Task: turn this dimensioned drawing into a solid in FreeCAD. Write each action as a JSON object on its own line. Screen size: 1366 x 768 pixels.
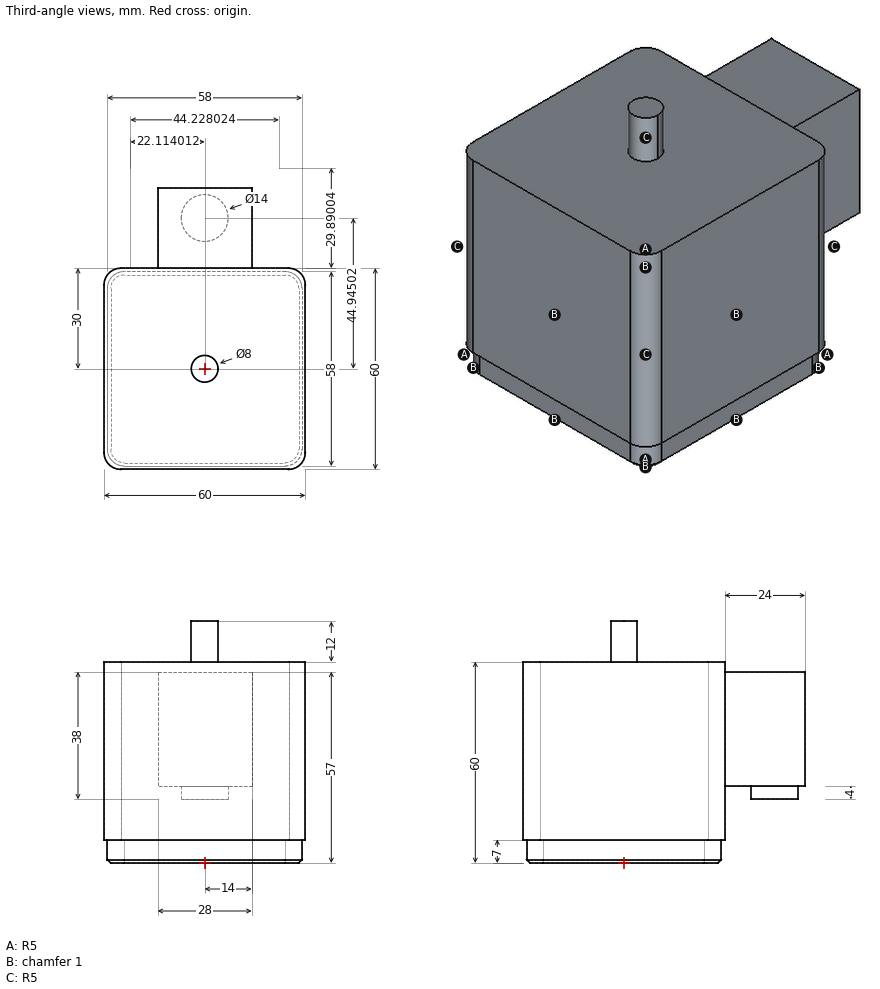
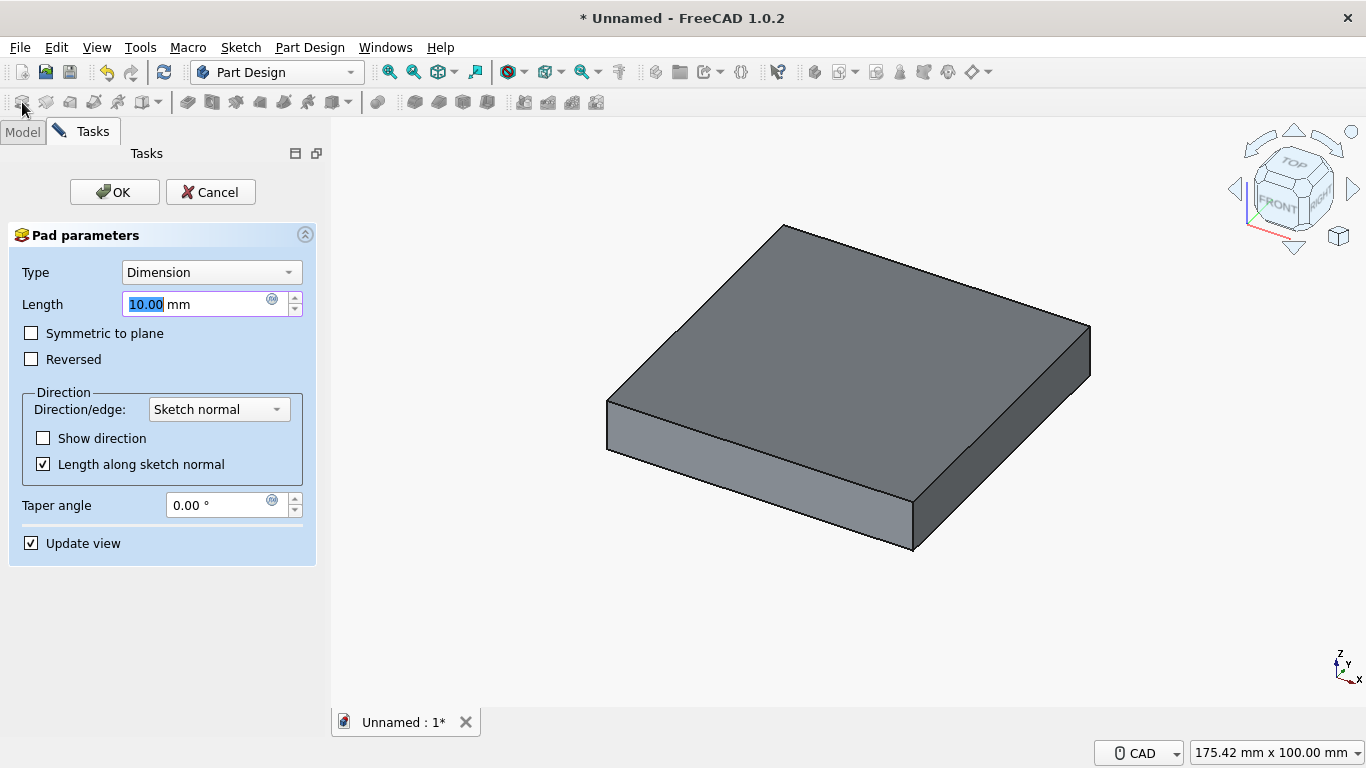
{"action": "type", "text": "60"}
{"action": "key", "text": "Tab"}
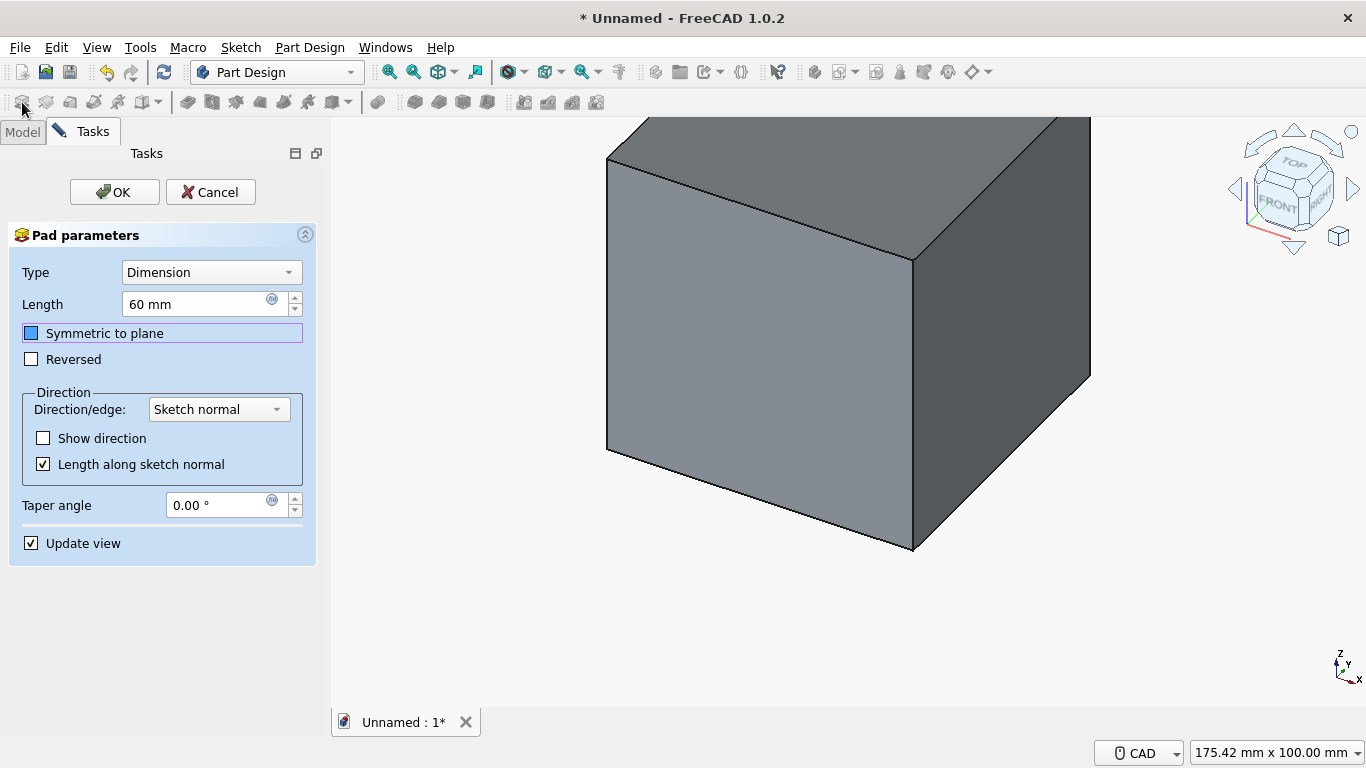
{"action": "left_click", "coordinate": [115, 192]}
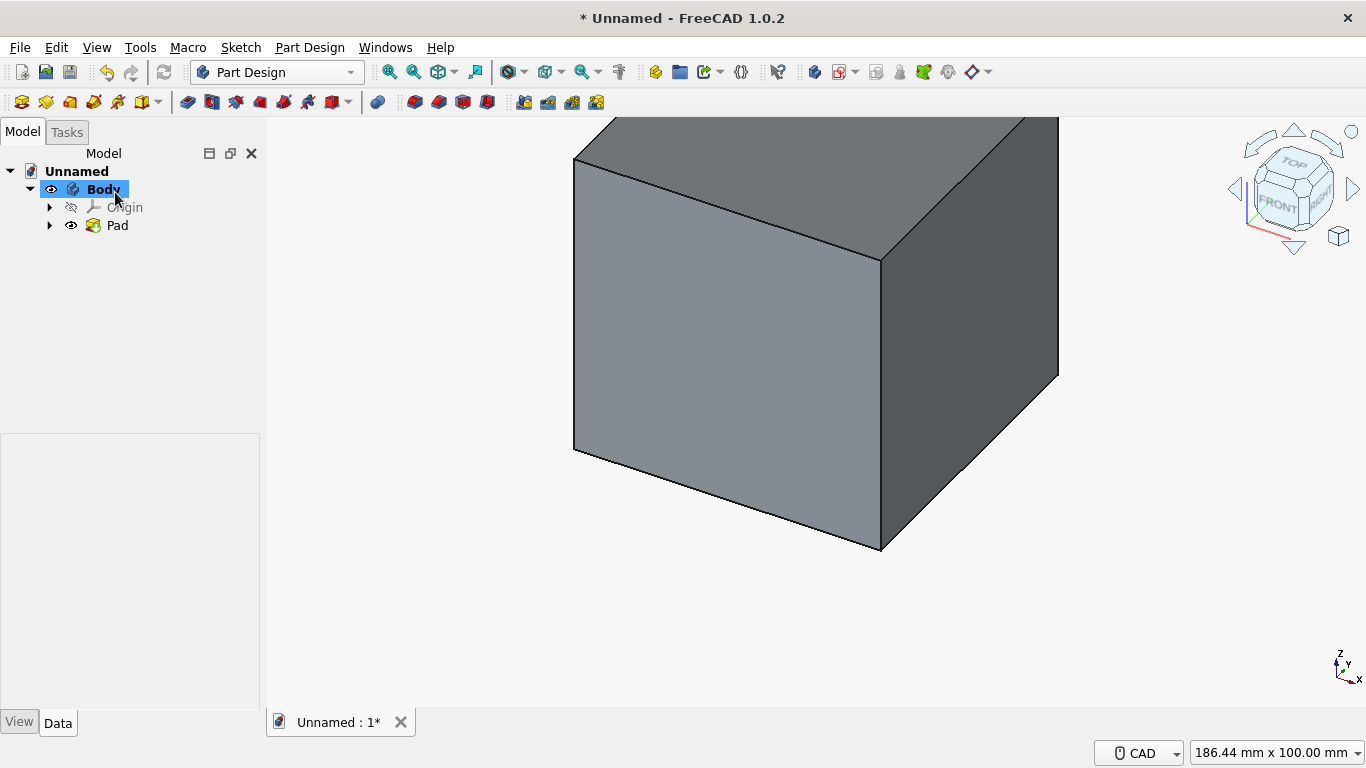
{"action": "key", "text": "v f"}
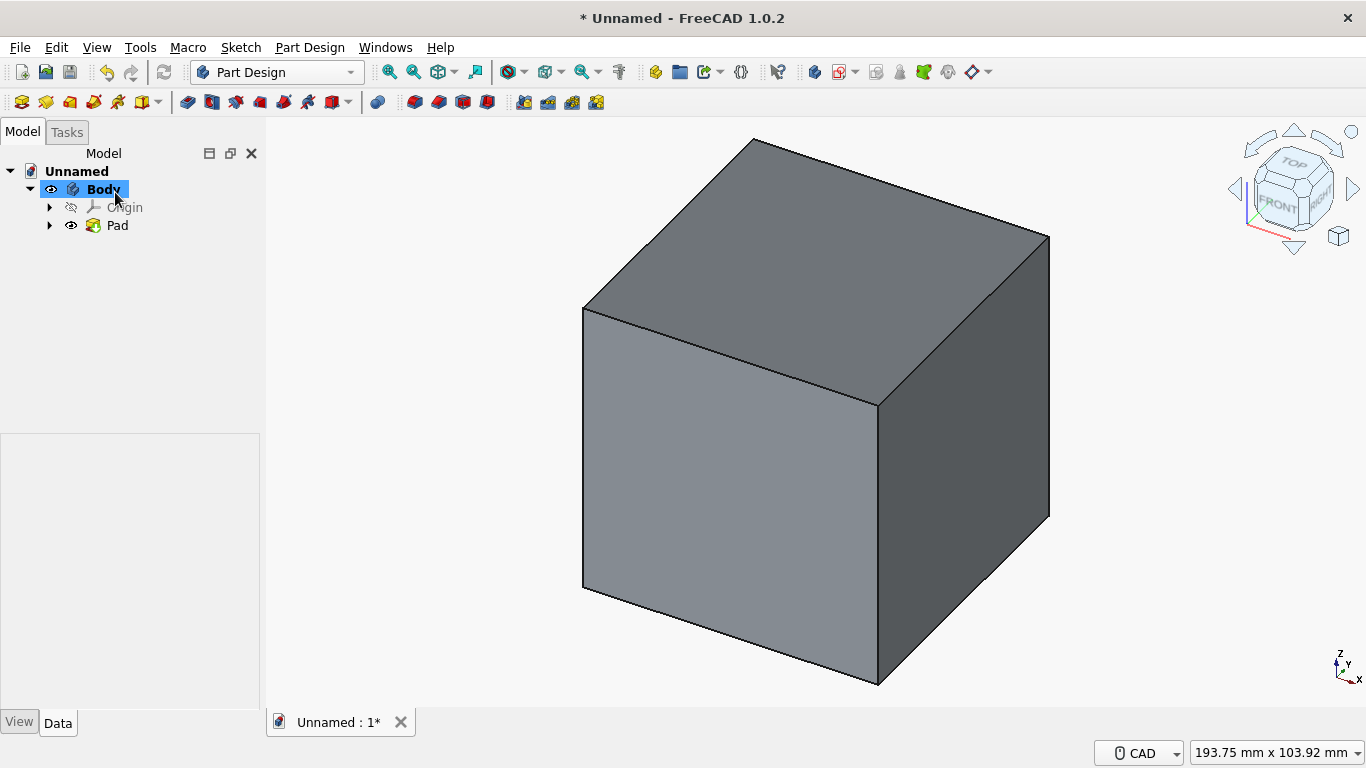
{"action": "left_click", "coordinate": [816, 271]}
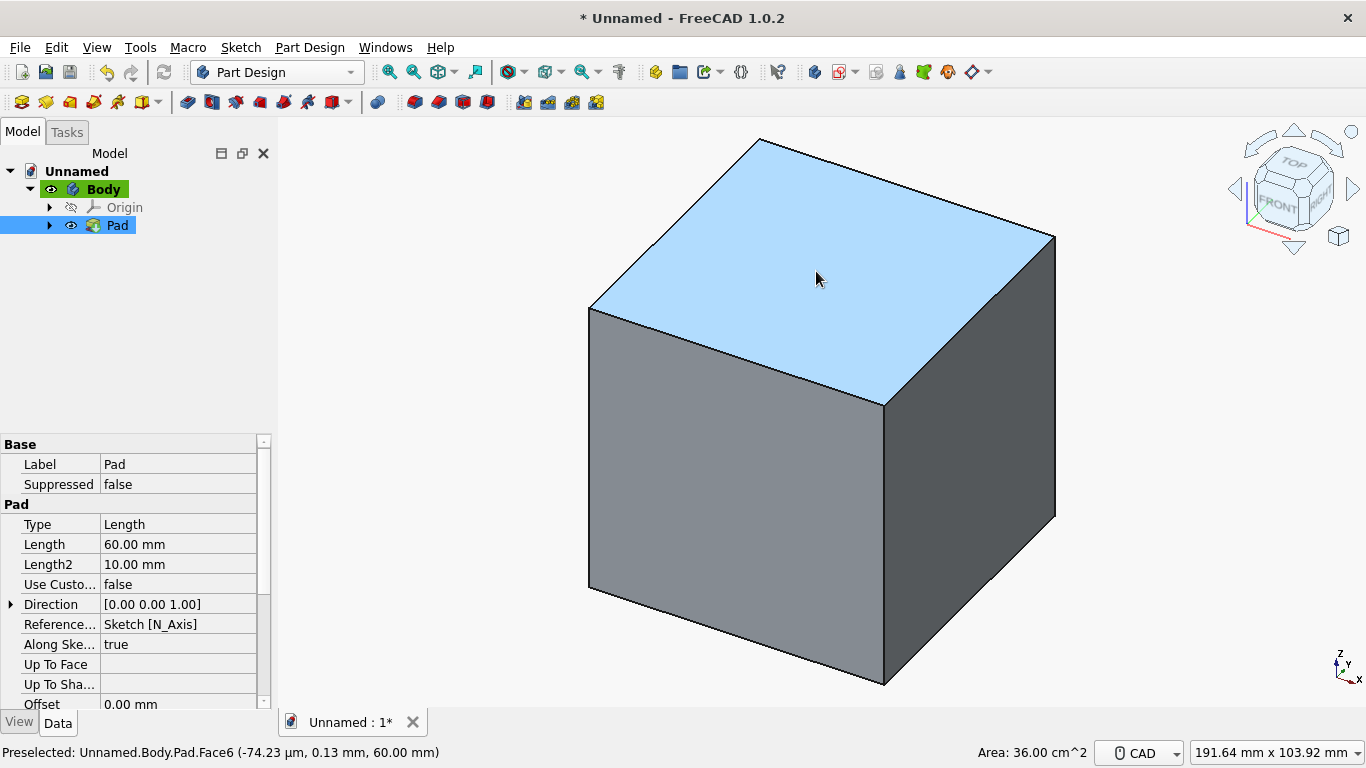
{"action": "left_click", "coordinate": [840, 72]}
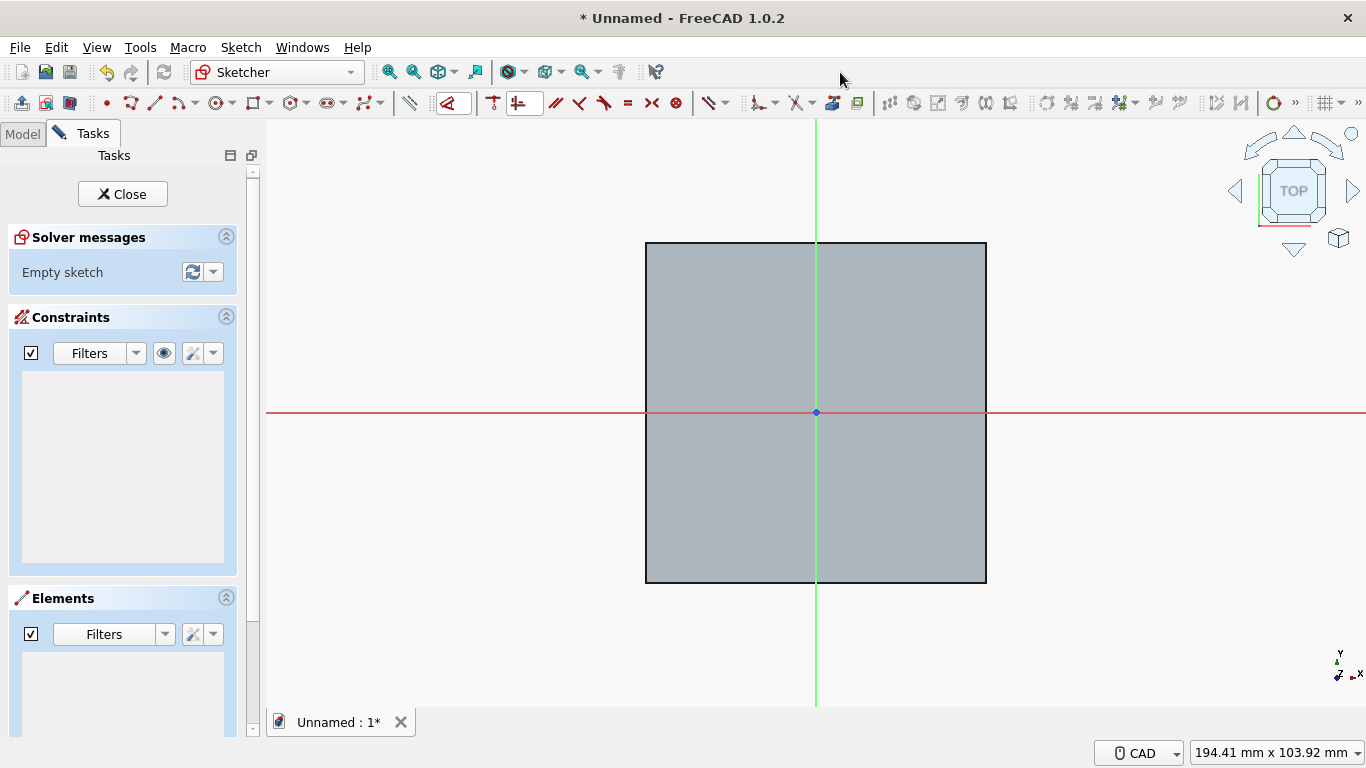
{"action": "scroll", "coordinate": [825, 413], "scroll_direction": "up", "scroll_amount": 11}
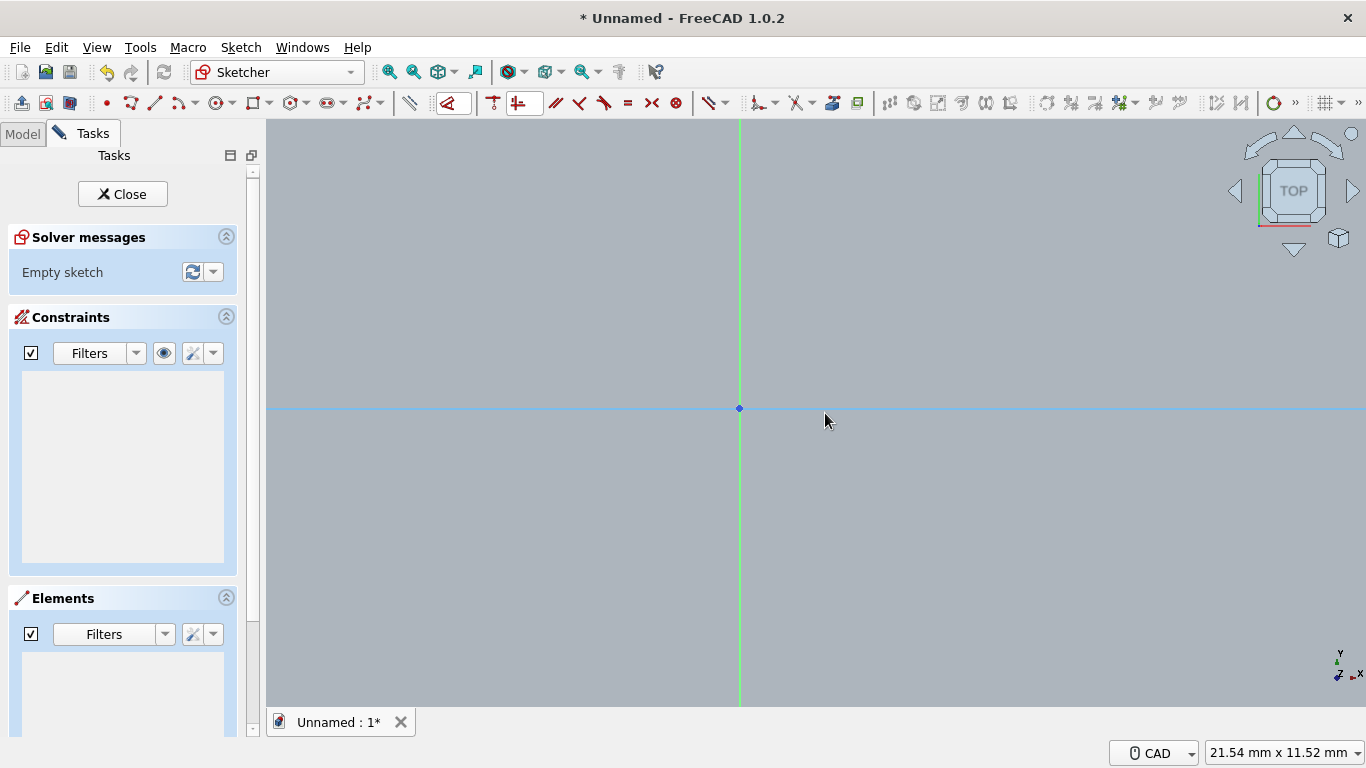
{"action": "left_click", "coordinate": [216, 104]}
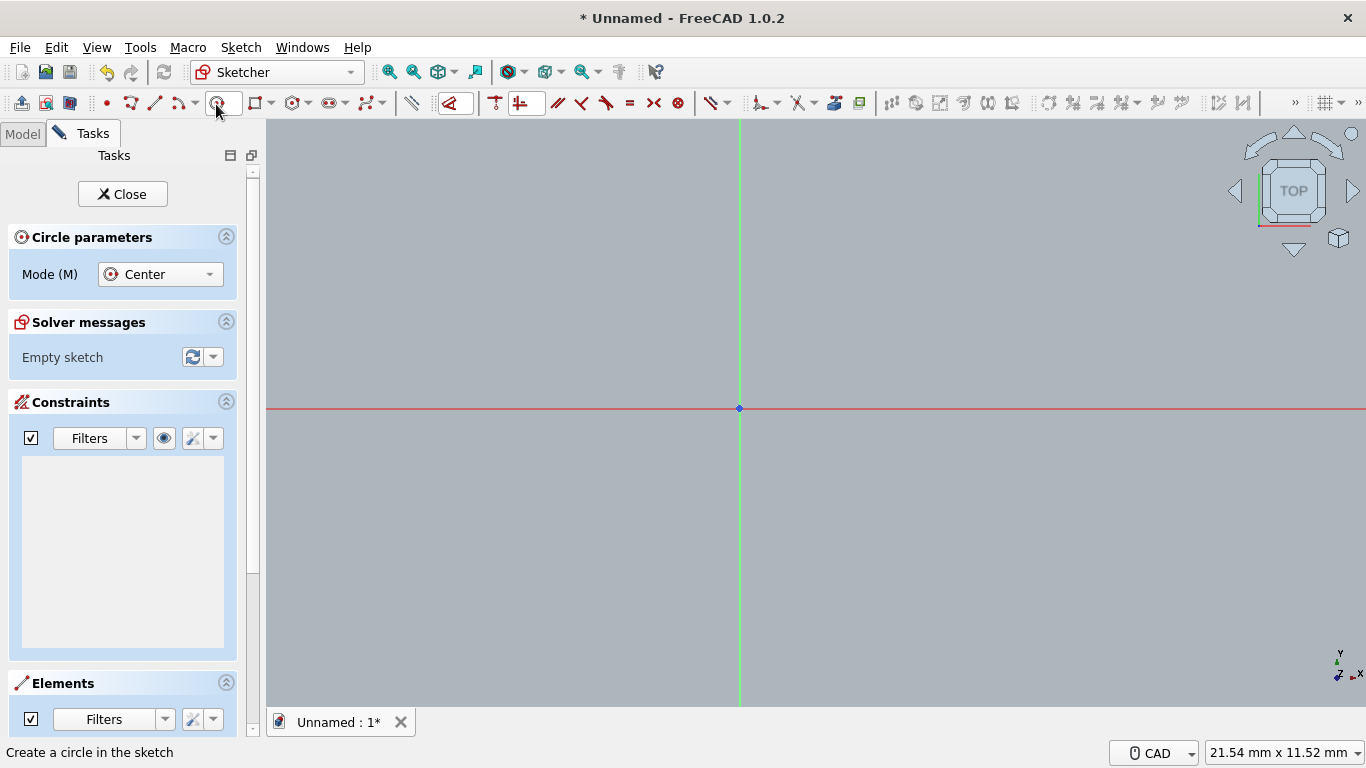
{"action": "left_click", "coordinate": [740, 409]}
{"action": "mouse_move", "coordinate": [884, 265]}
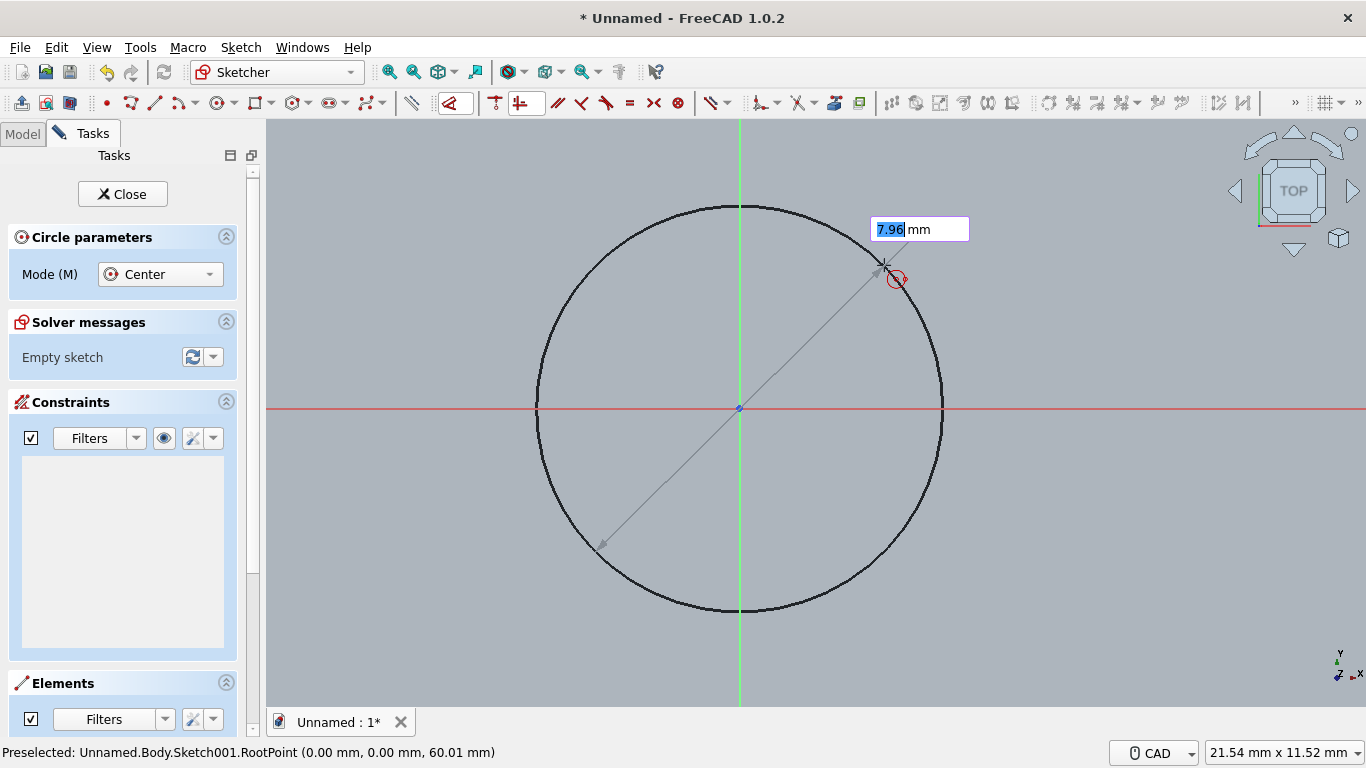
{"action": "type", "text": "8"}
{"action": "key", "text": "Return"}
{"action": "key", "text": "Escape"}